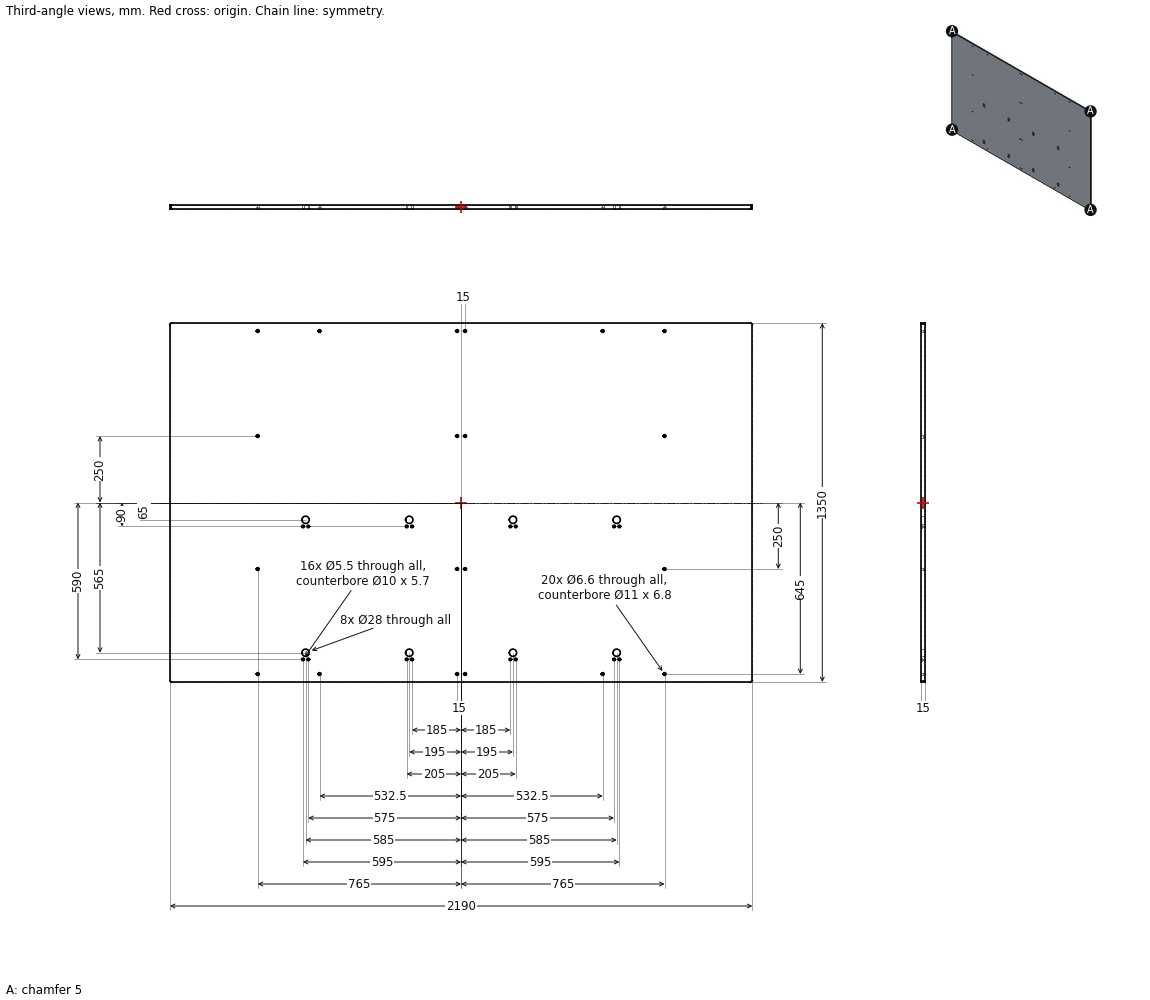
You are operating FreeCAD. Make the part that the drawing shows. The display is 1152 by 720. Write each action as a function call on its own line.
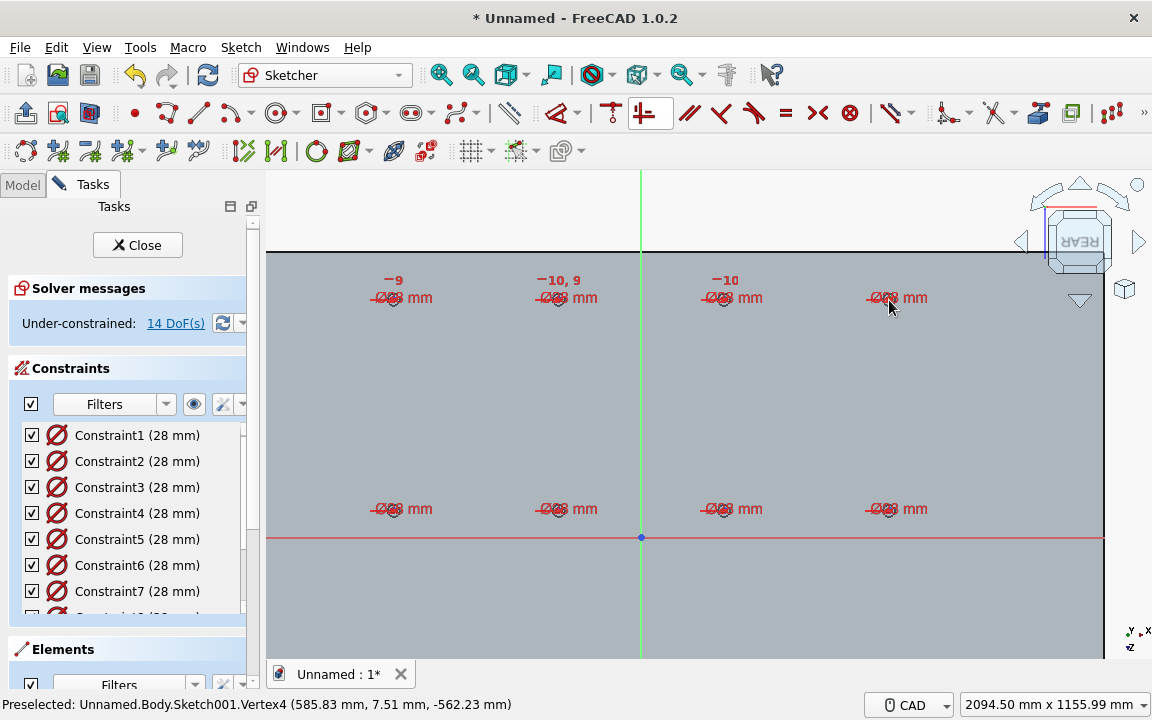
key(h)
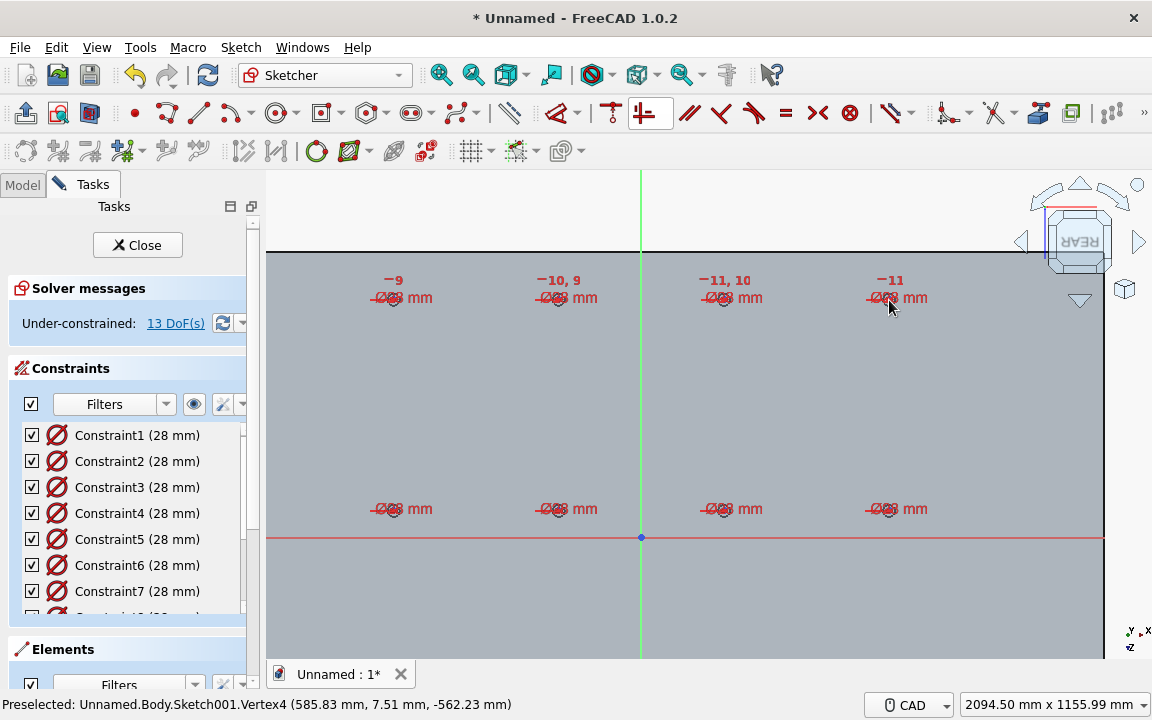
click(394, 300)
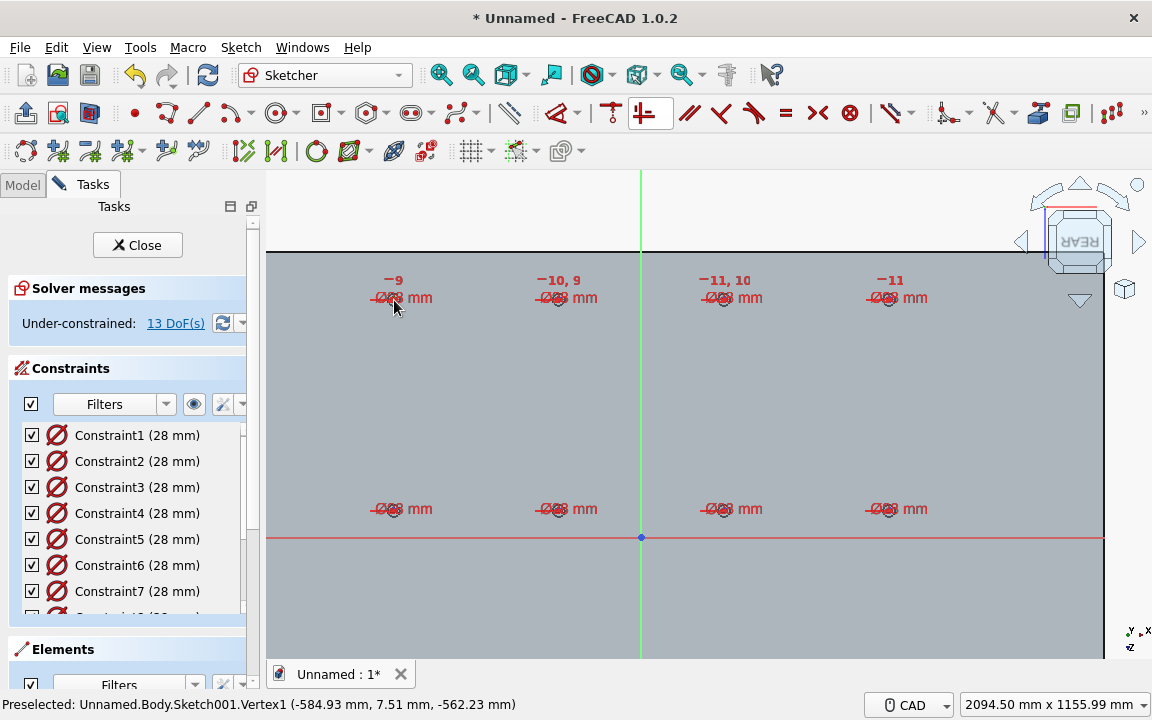
click(394, 511)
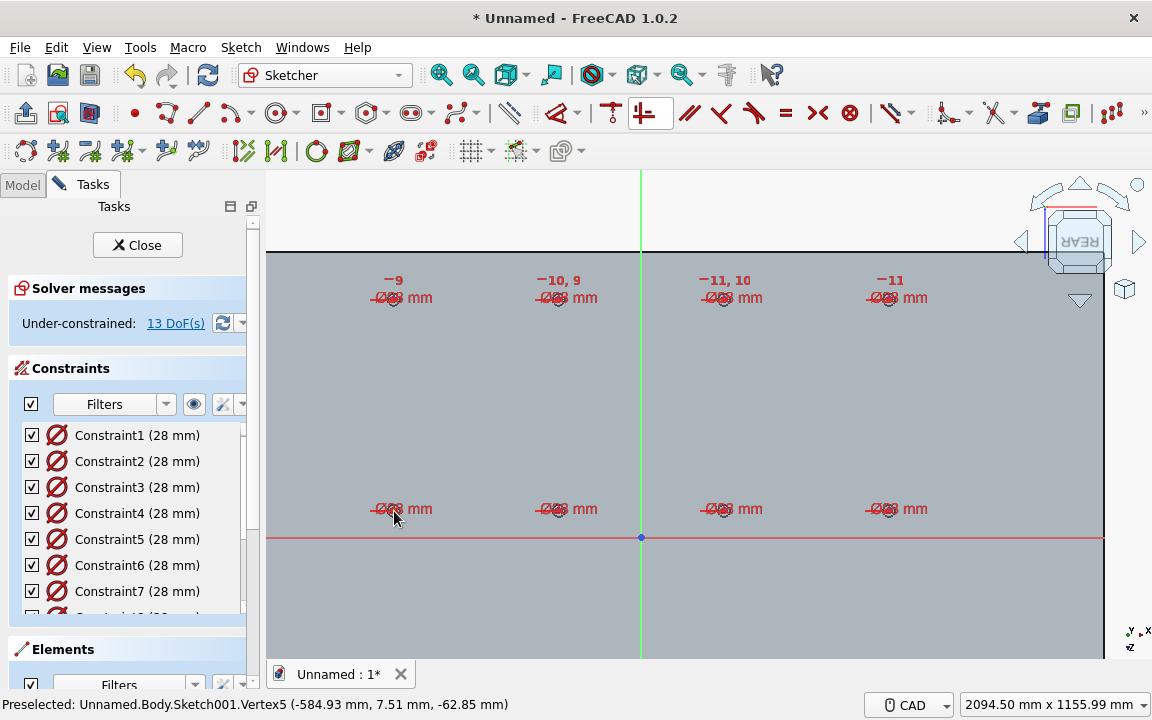
key(v)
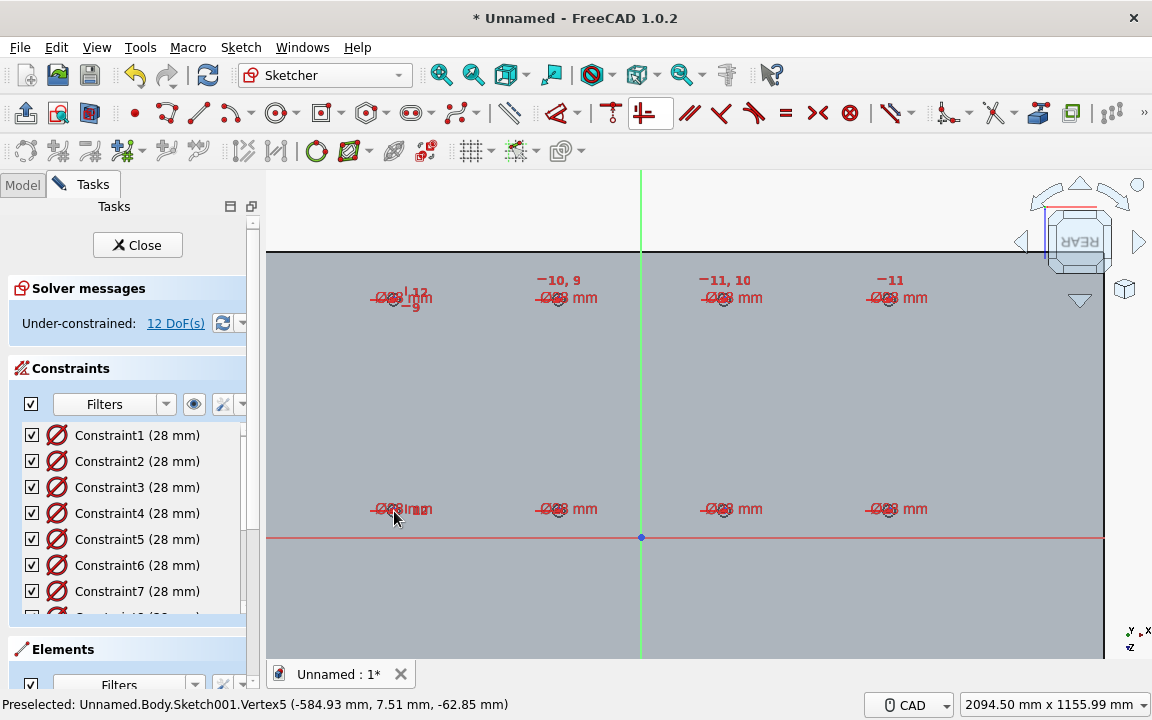
click(559, 300)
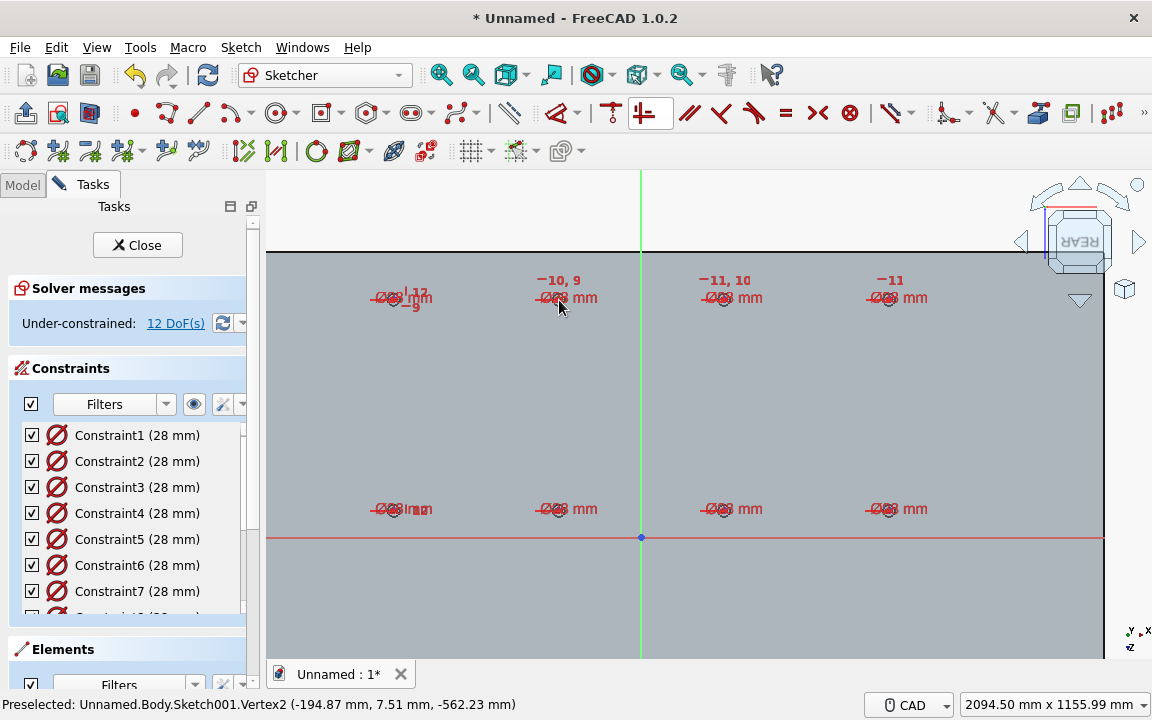
click(559, 511)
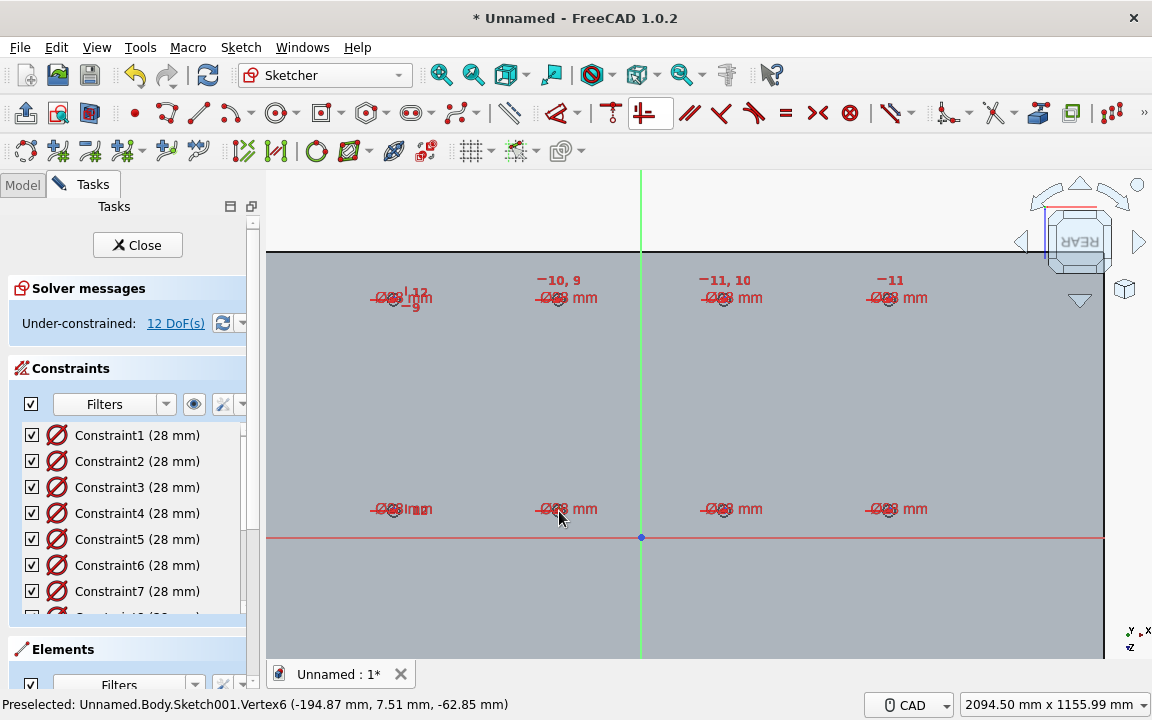
key(v)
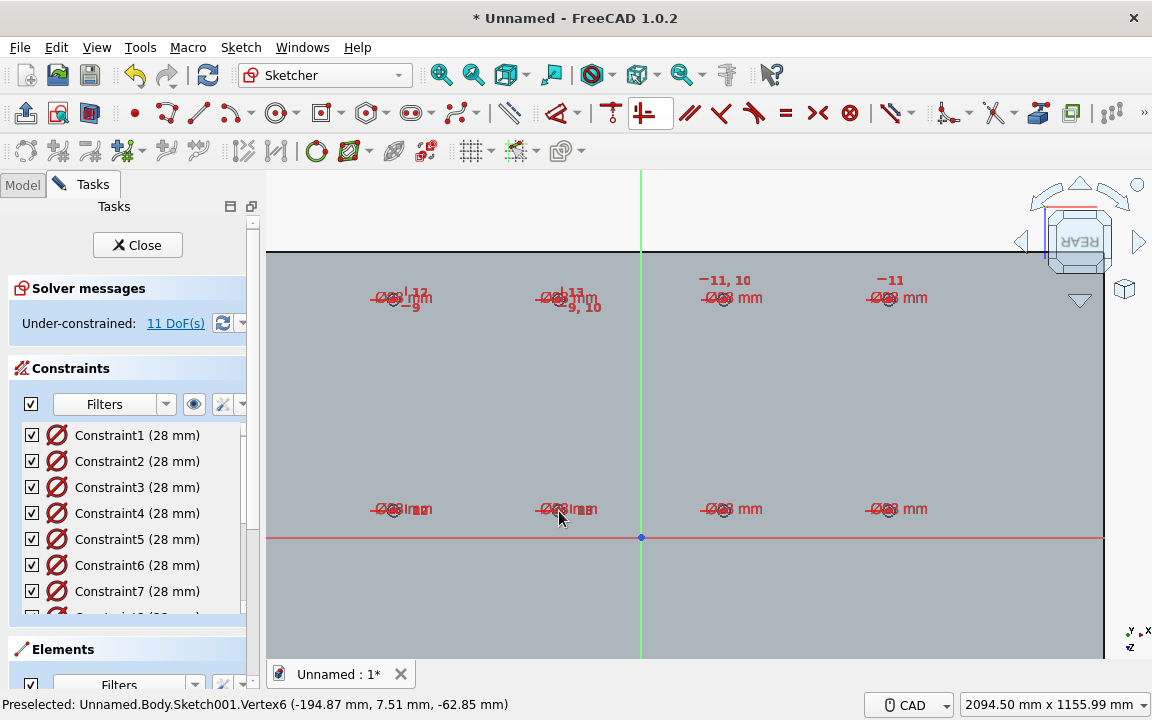
click(394, 511)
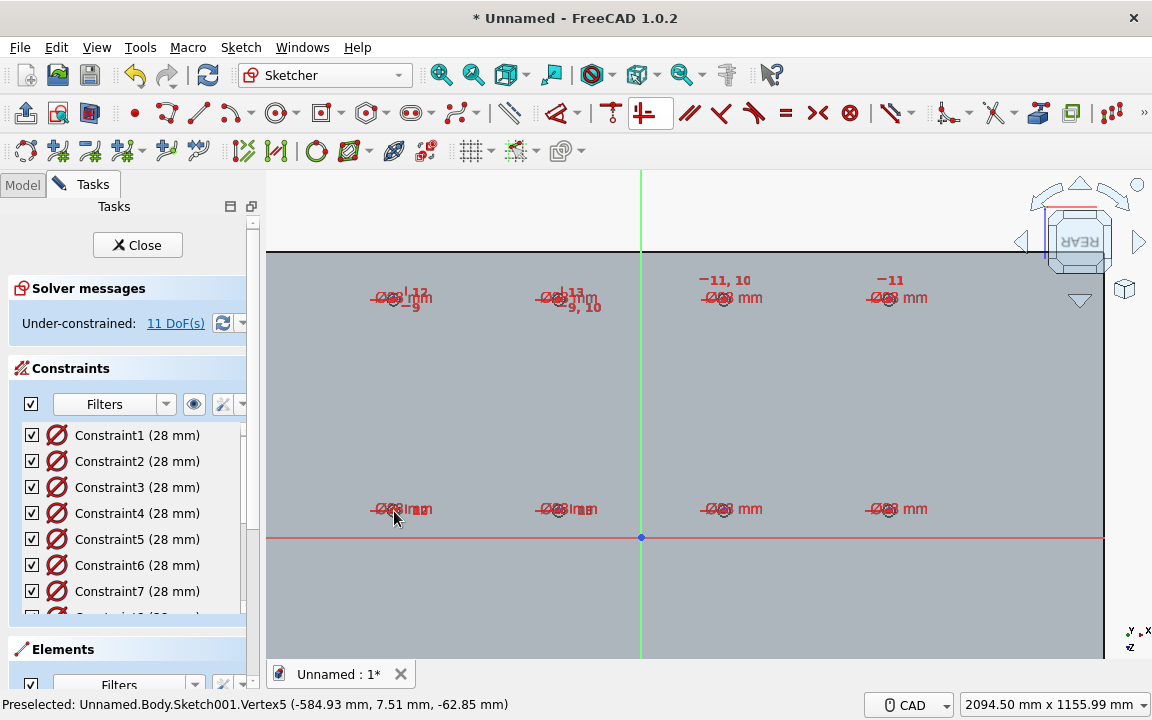
click(559, 511)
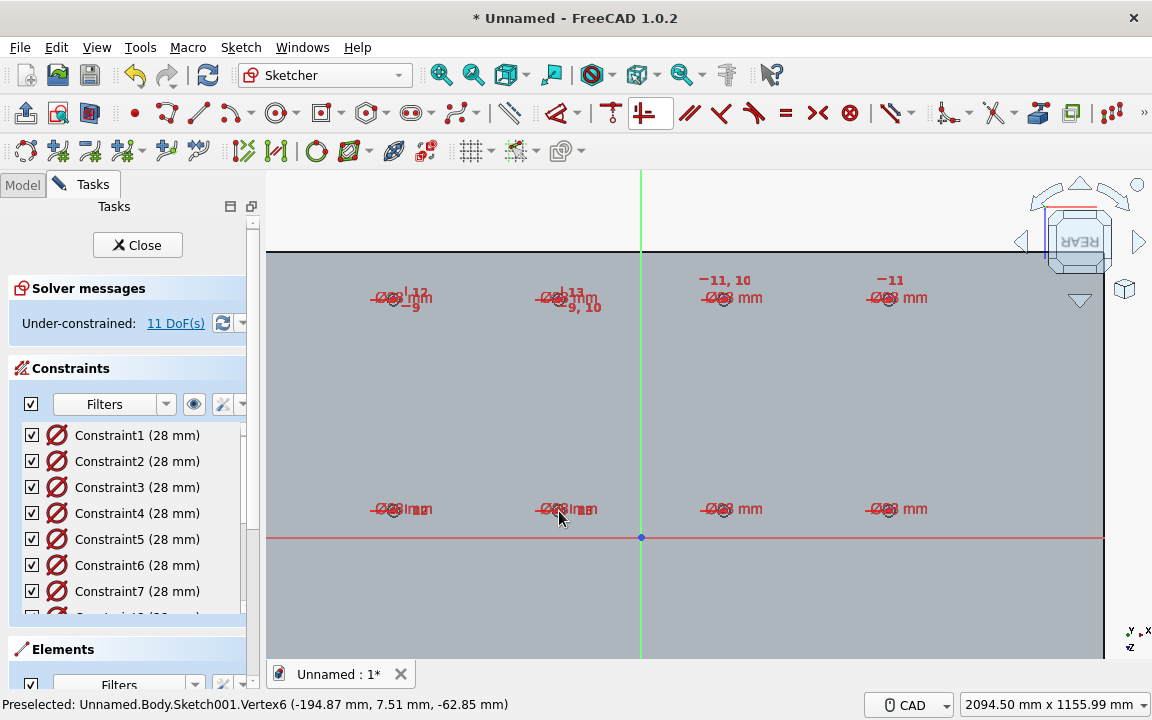
key(h)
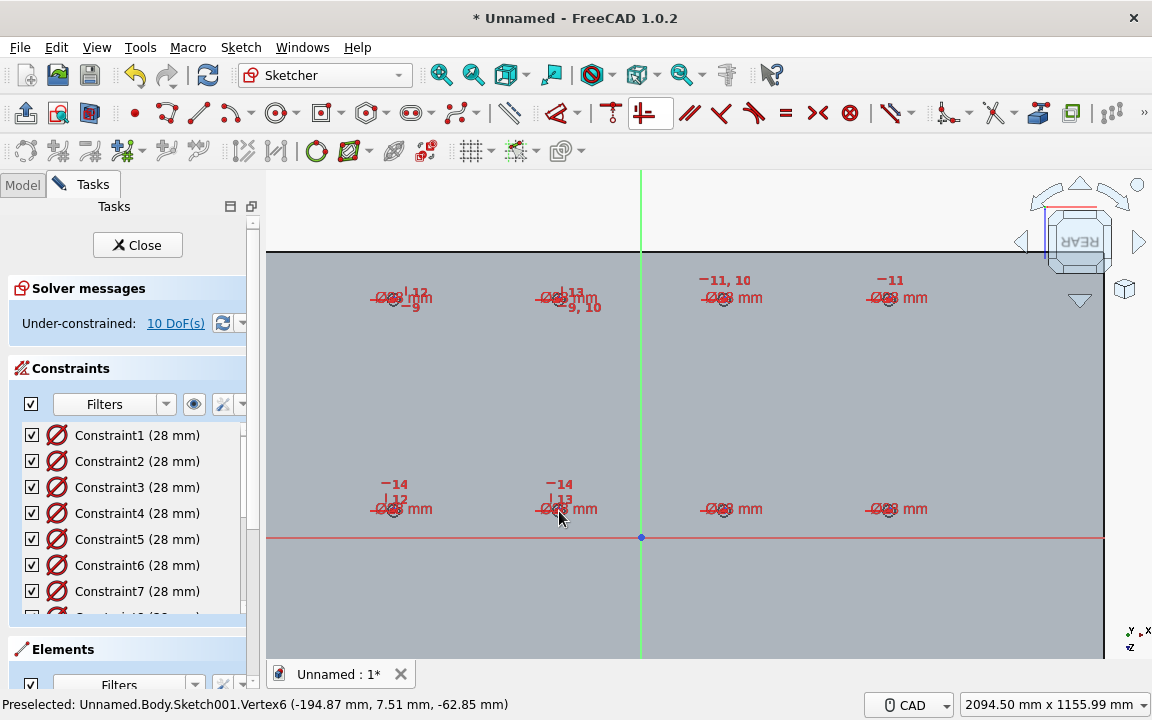
click(724, 300)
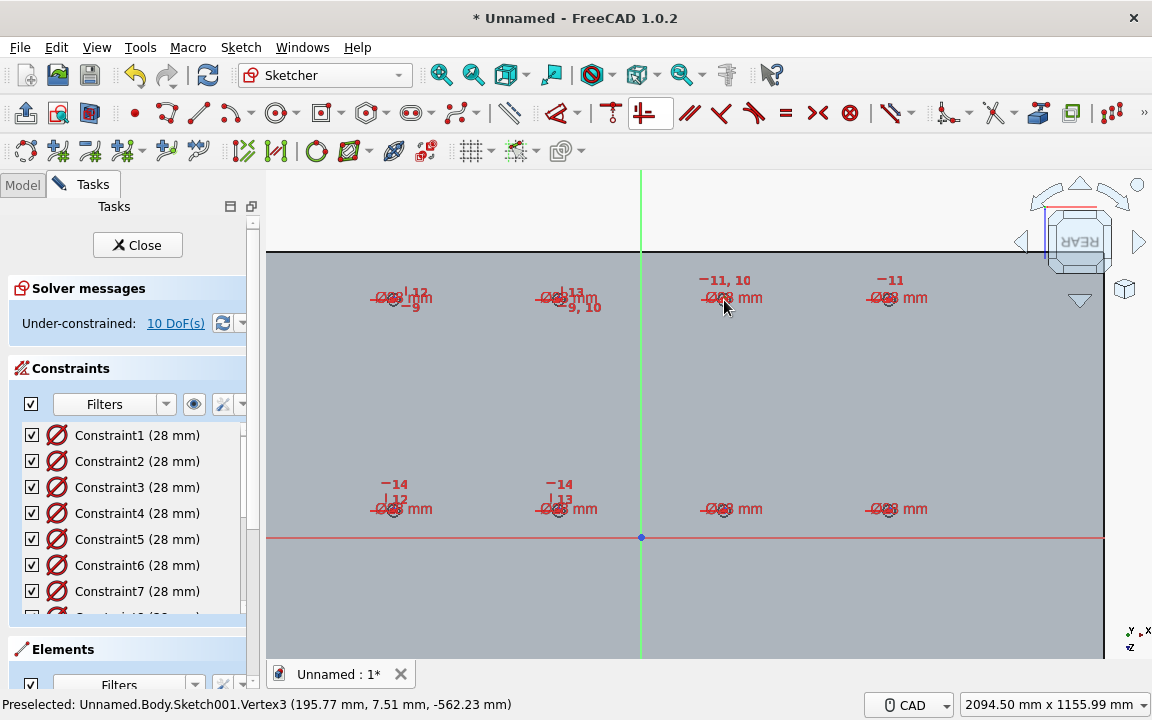
click(724, 511)